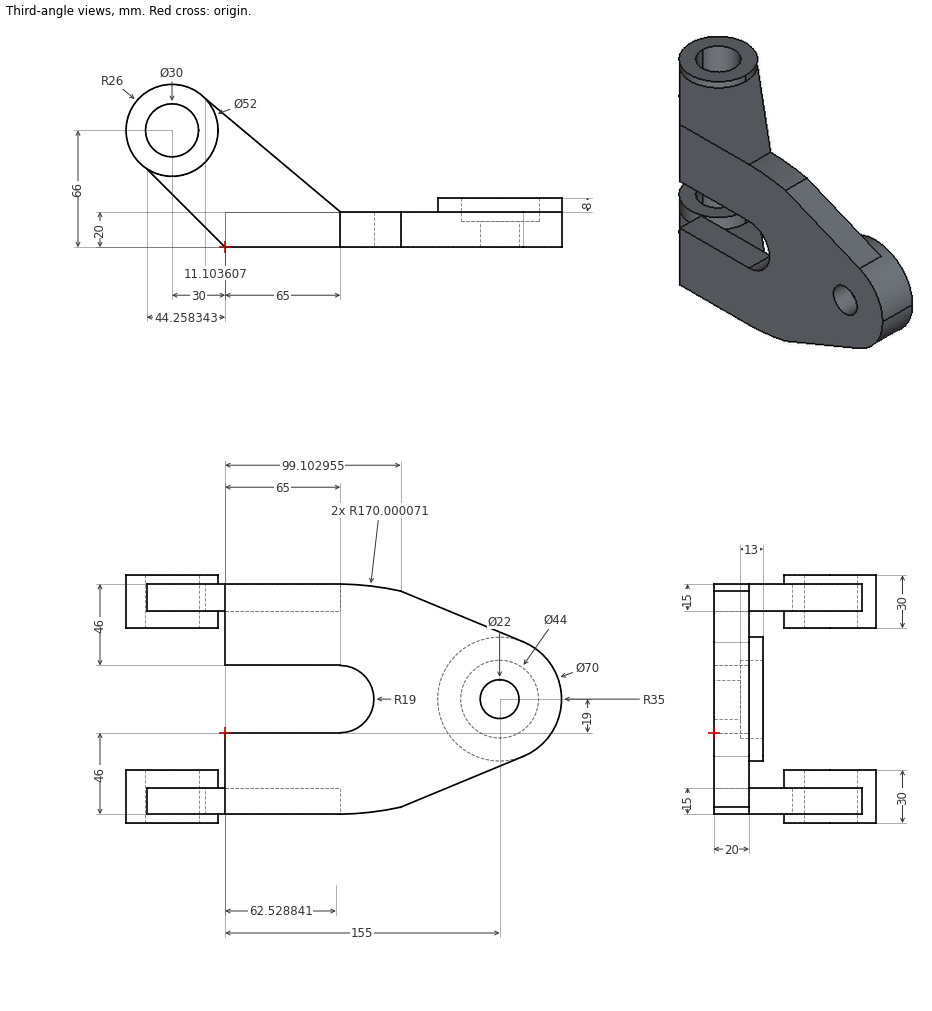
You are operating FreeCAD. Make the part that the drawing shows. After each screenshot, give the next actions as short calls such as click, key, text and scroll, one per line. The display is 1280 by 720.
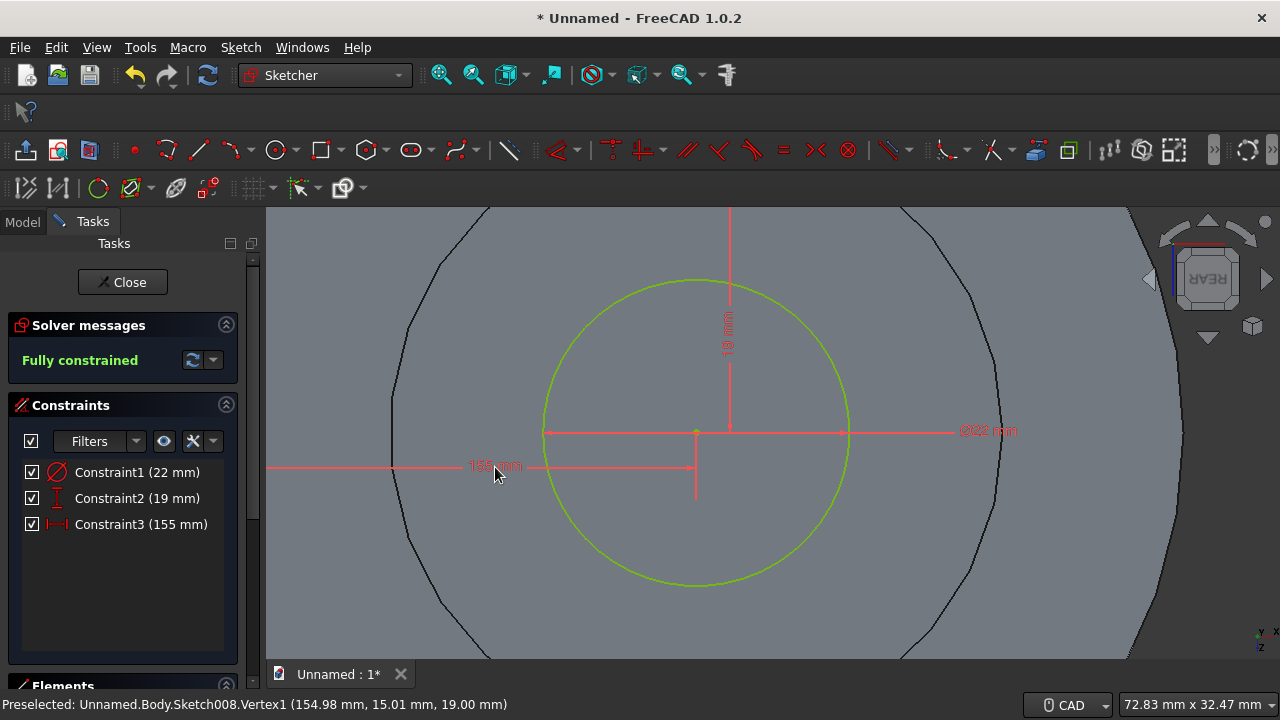
click(123, 282)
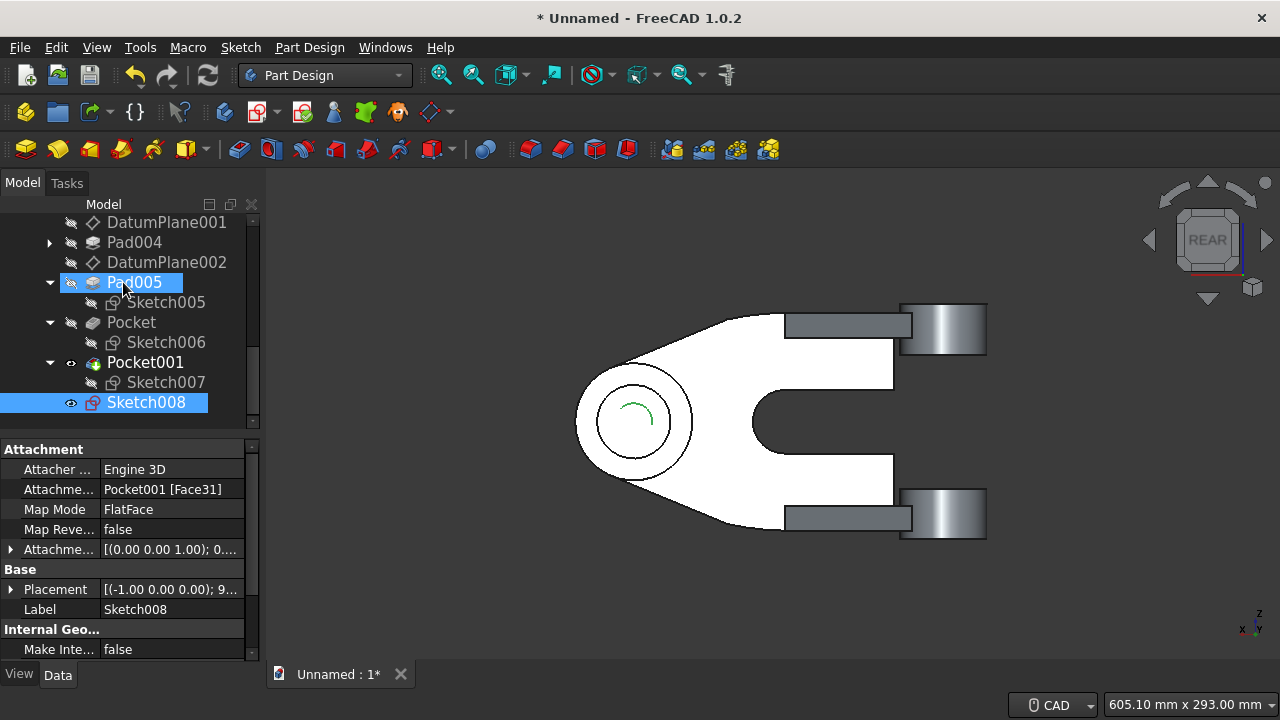
click(240, 150)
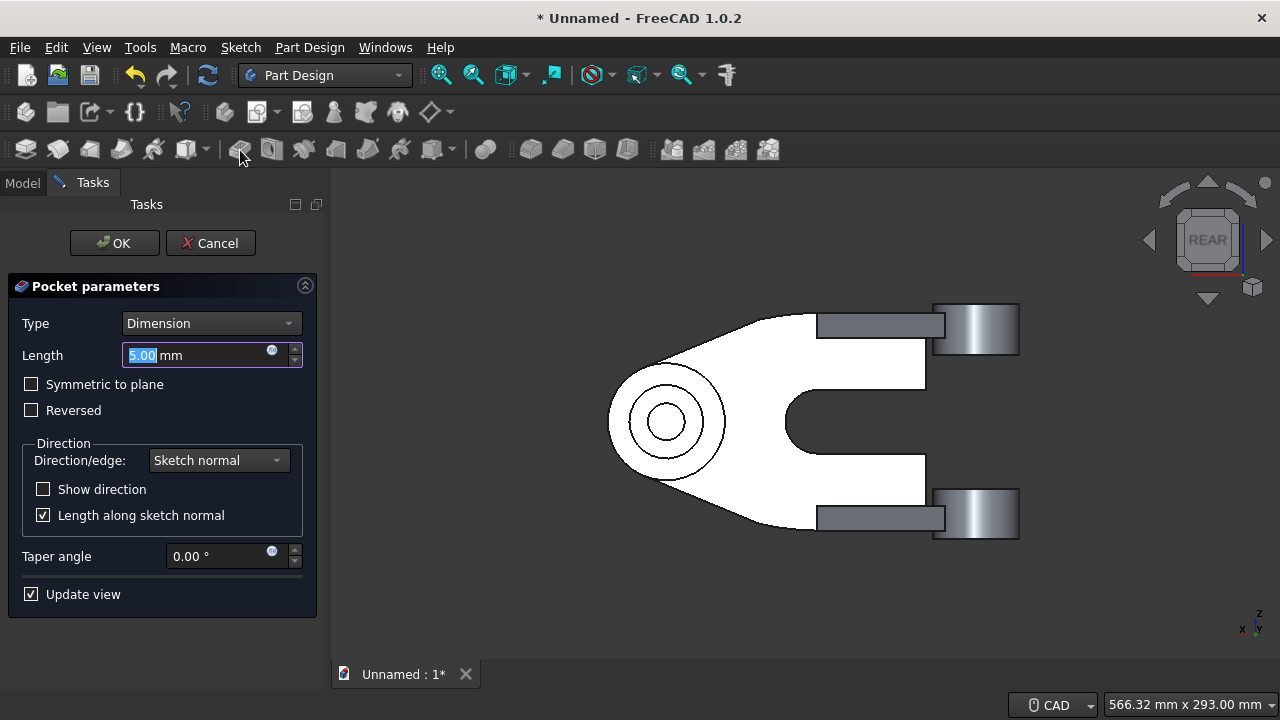
click(212, 324)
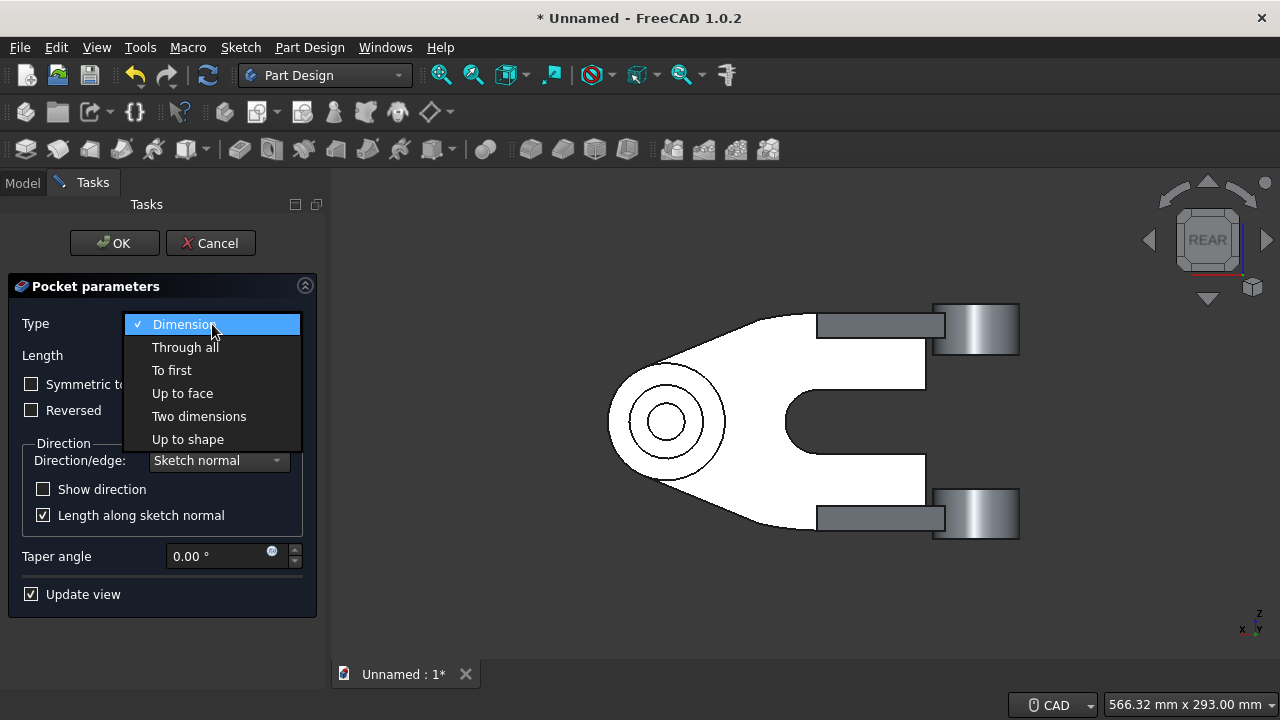
click(212, 348)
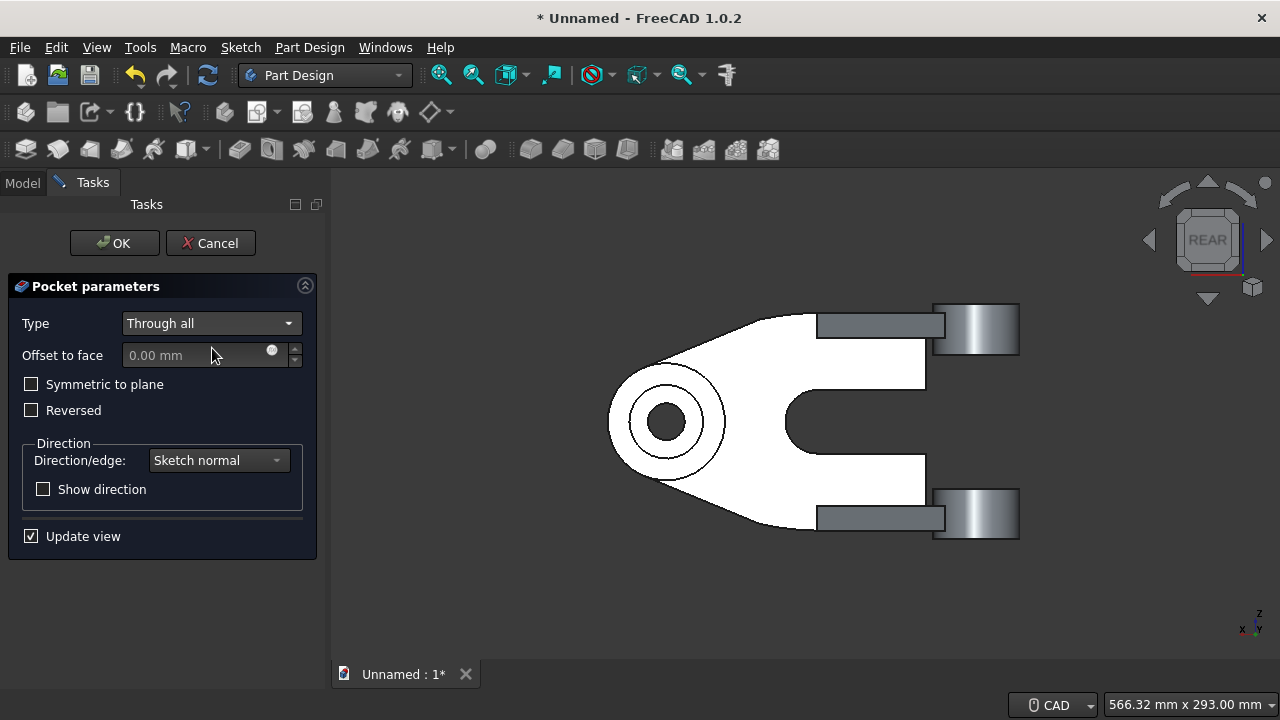
click(115, 243)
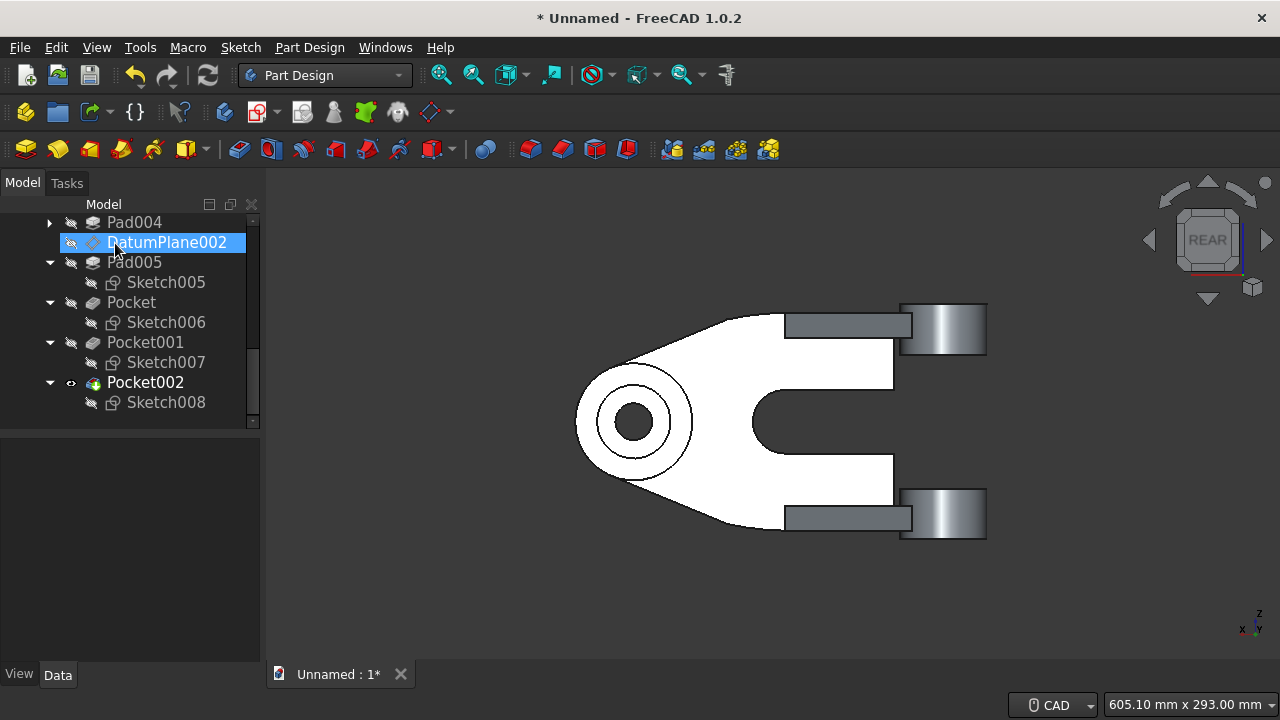
key(0)